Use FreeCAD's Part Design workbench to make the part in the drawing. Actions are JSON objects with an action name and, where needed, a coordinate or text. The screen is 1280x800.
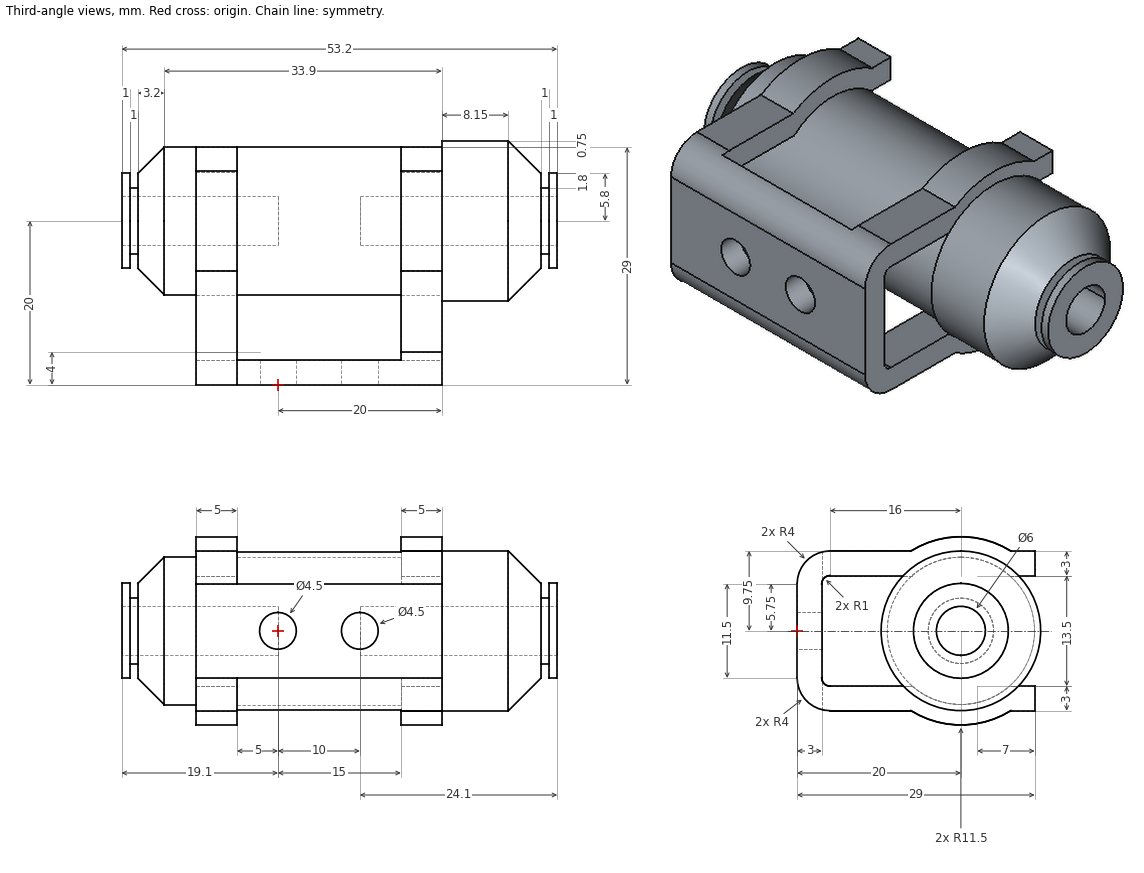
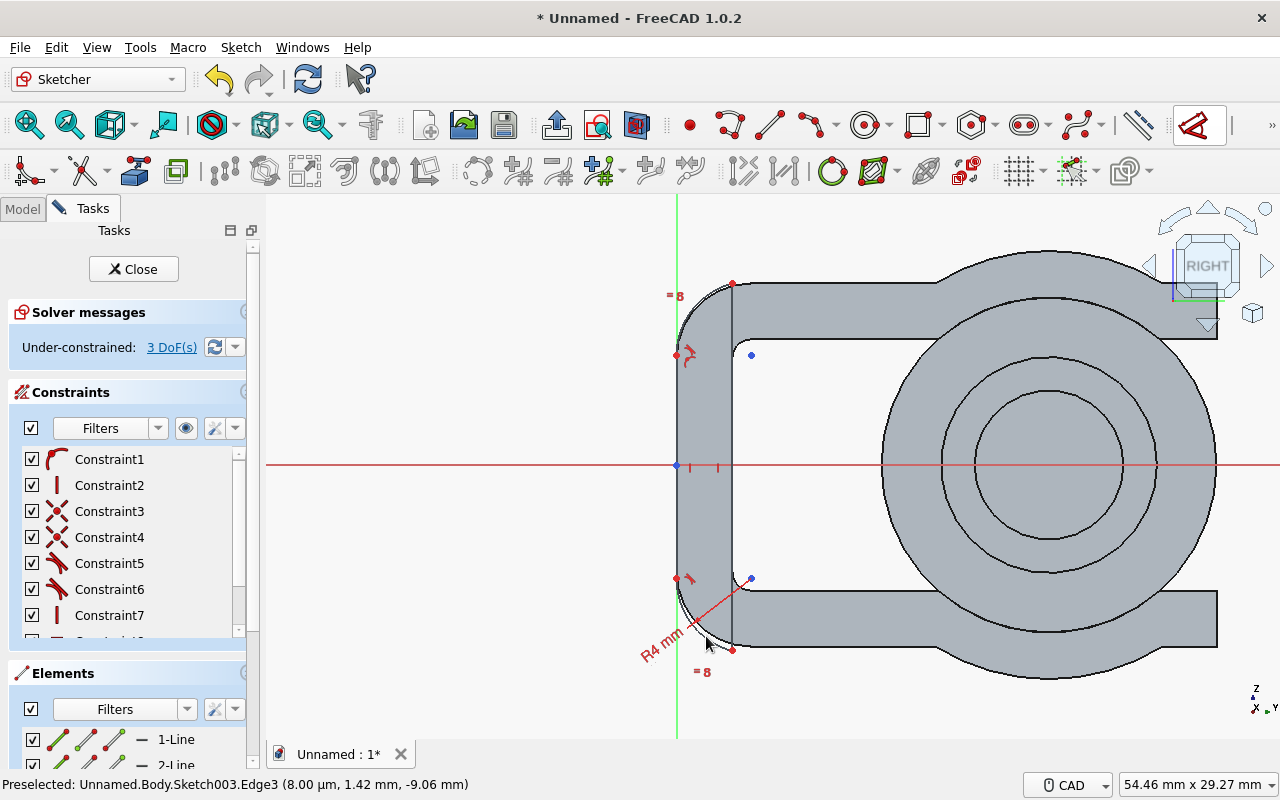
{"action": "left_click", "coordinate": [732, 651]}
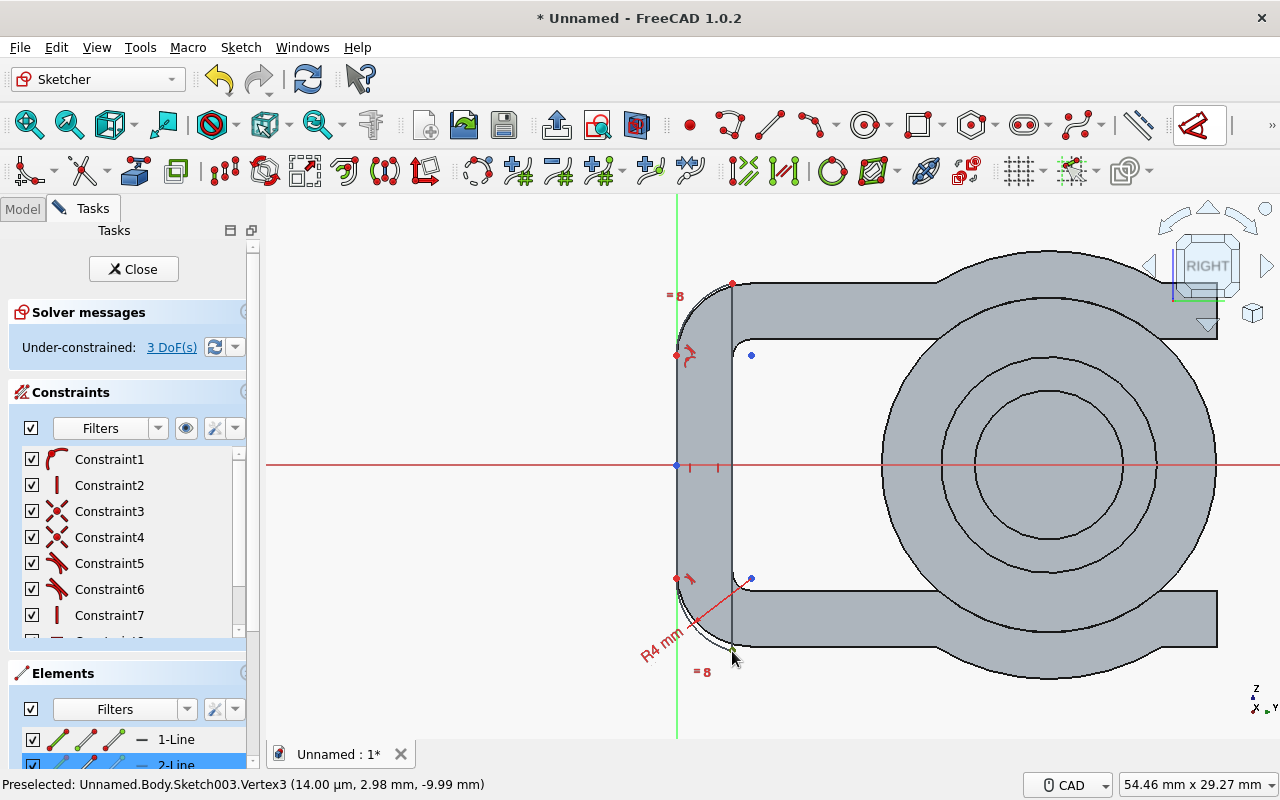
{"action": "key", "text": "l"}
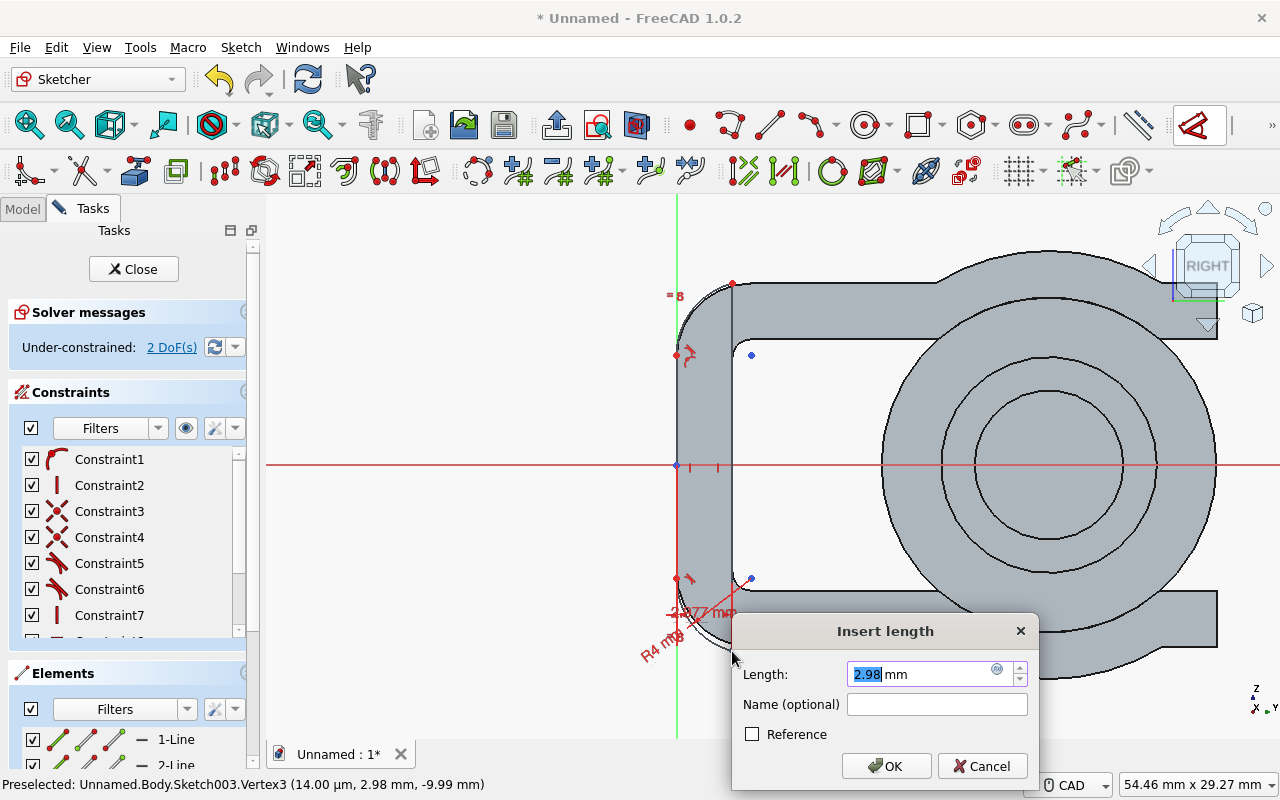
{"action": "type", "text": "3"}
{"action": "key", "text": "Return"}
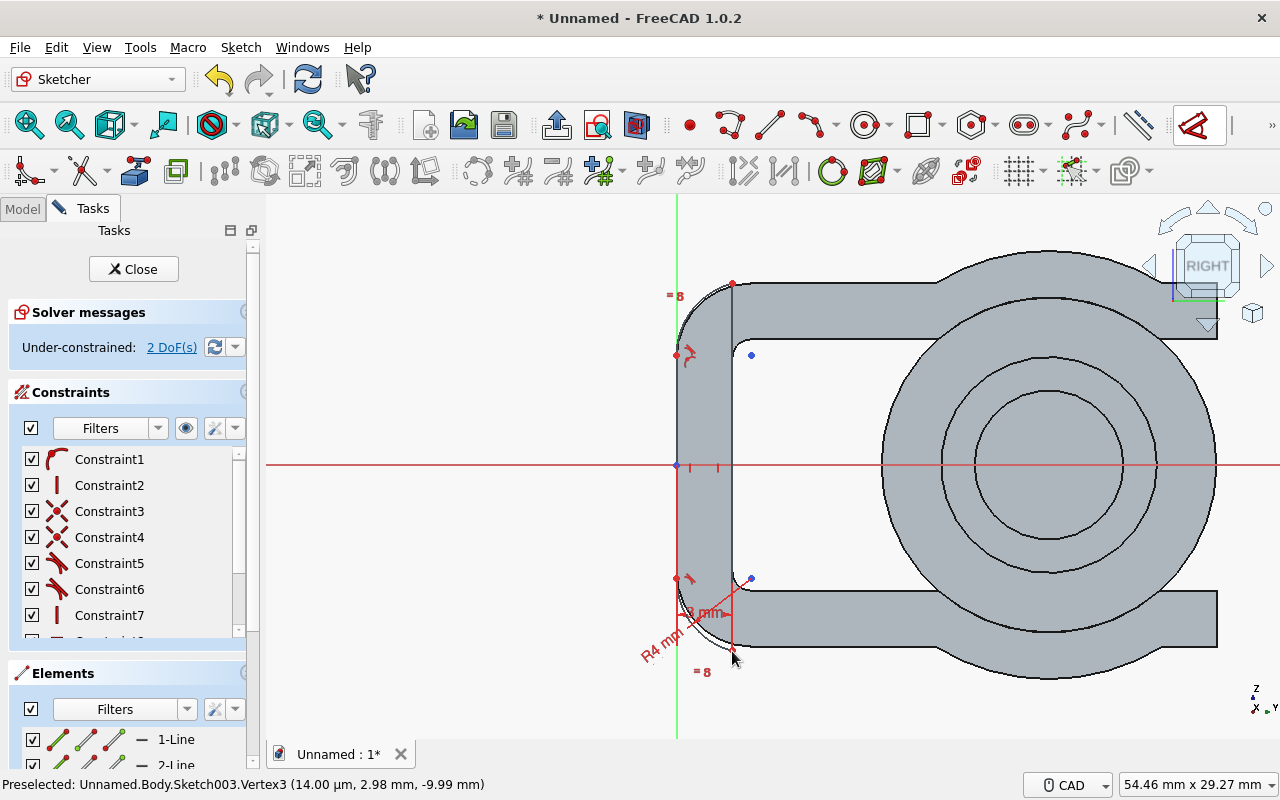
{"action": "left_click", "coordinate": [677, 423]}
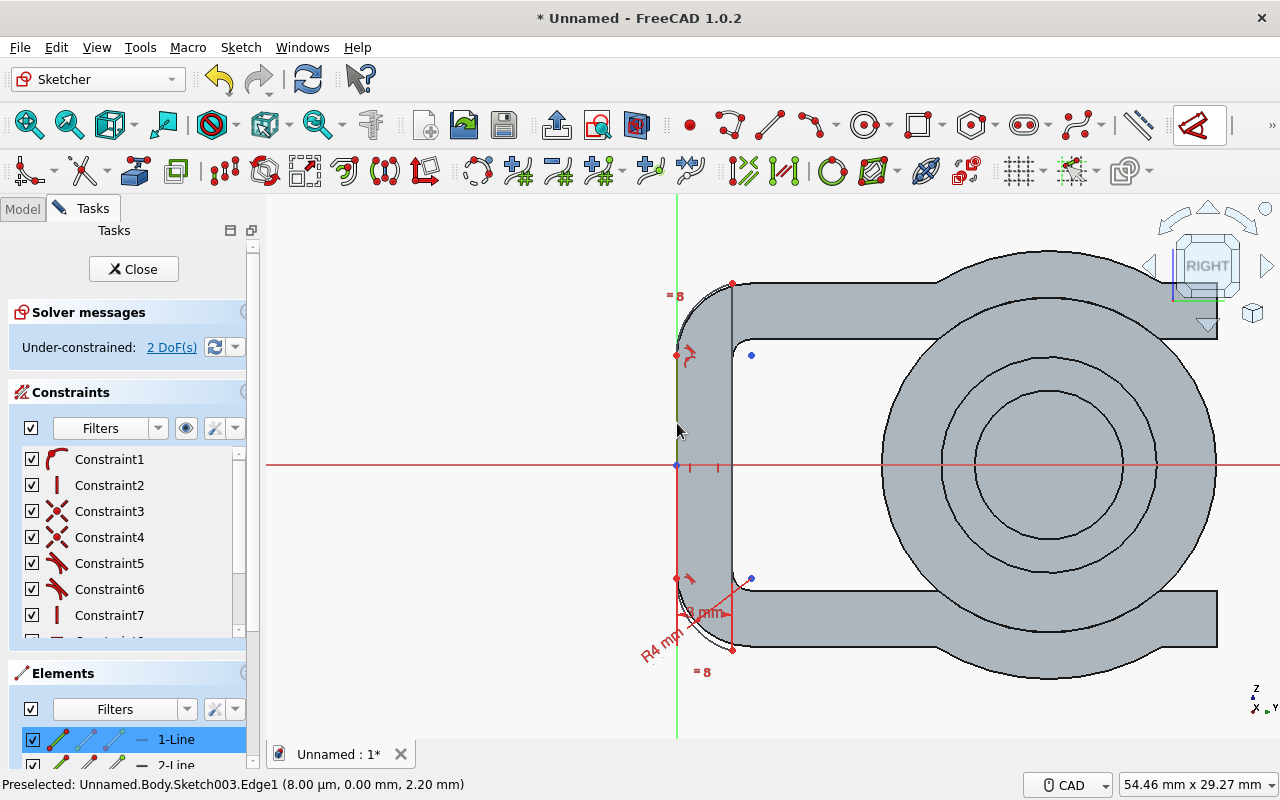
{"action": "key", "text": "i"}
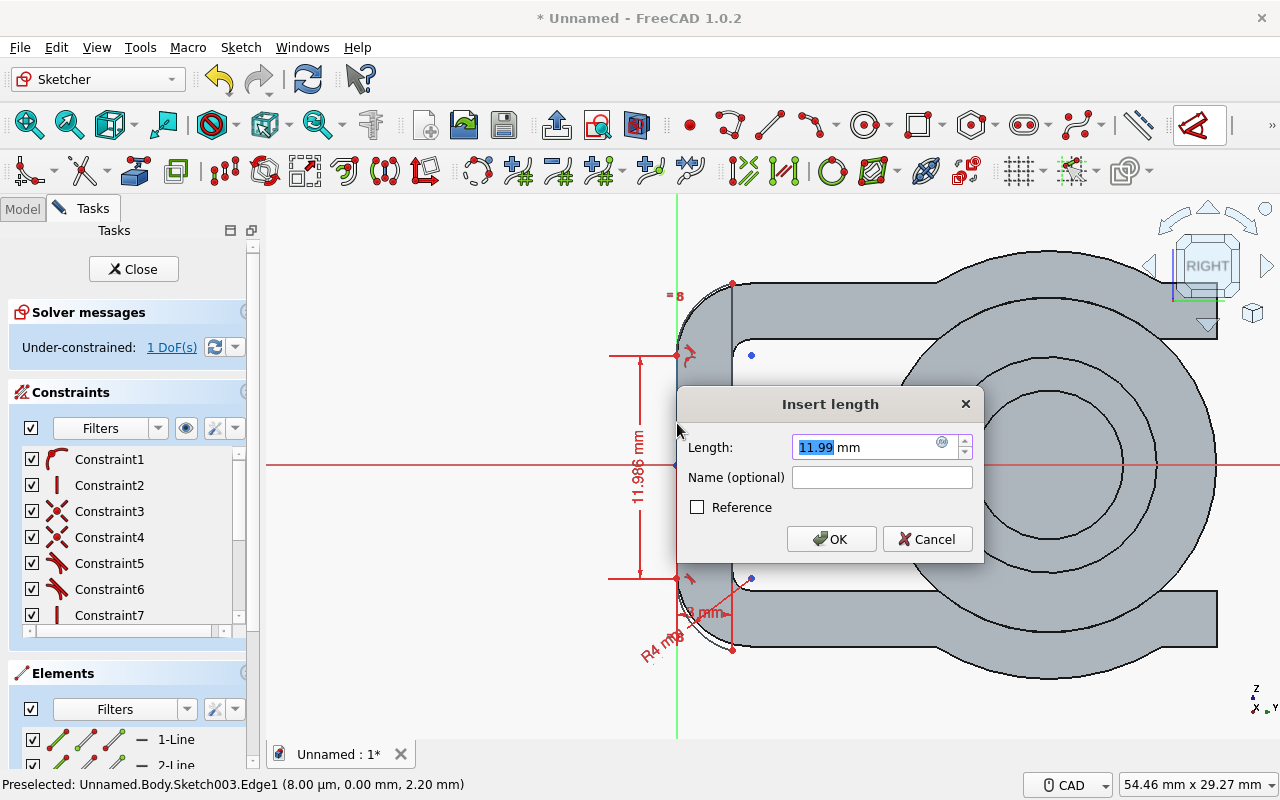
{"action": "type", "text": "11.5"}
{"action": "key", "text": "Return"}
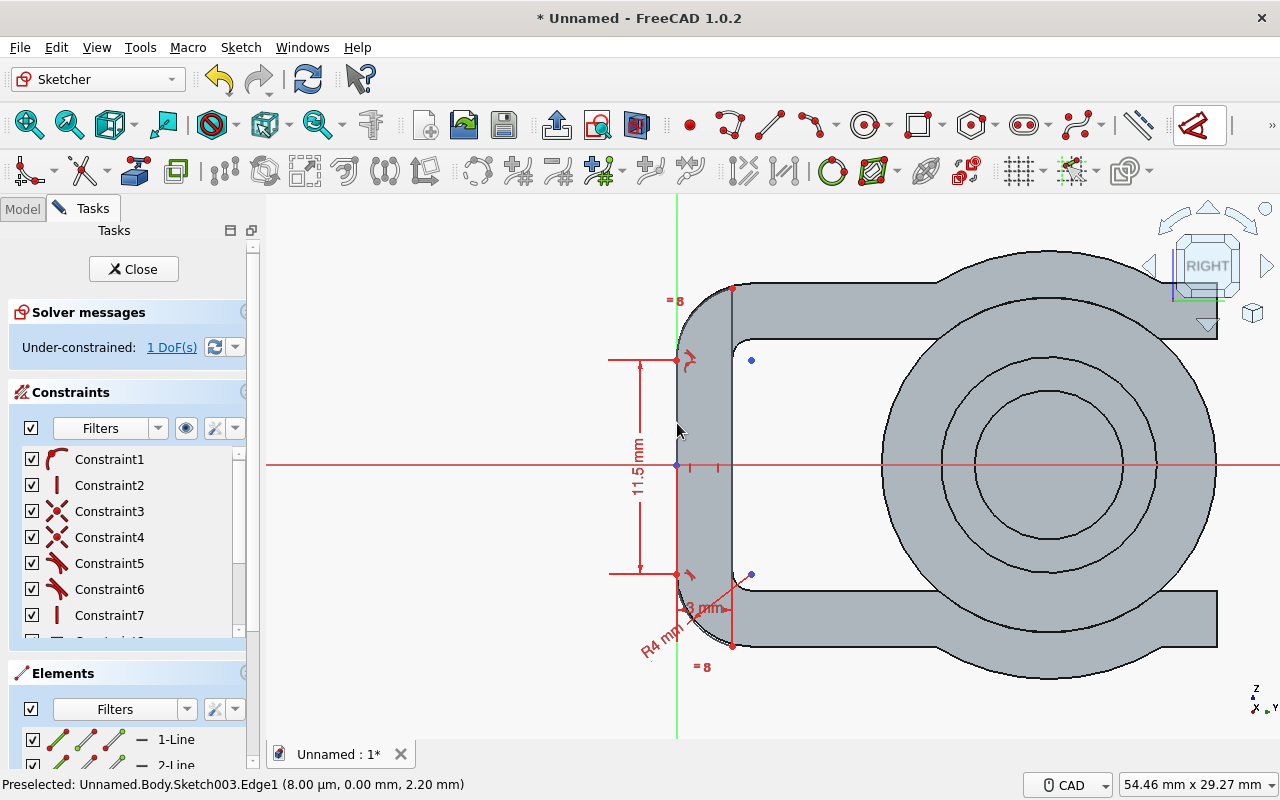
{"action": "left_click", "coordinate": [677, 360]}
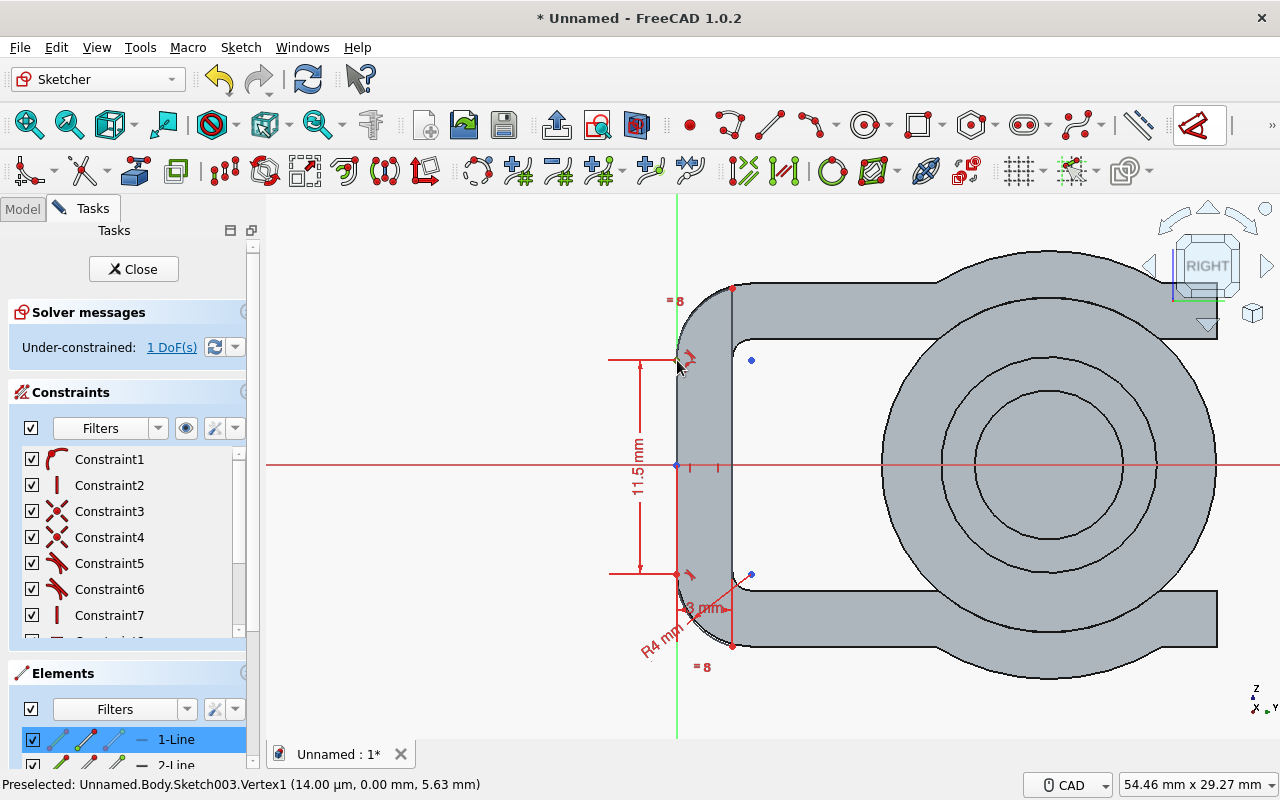
{"action": "left_click", "coordinate": [1220, 126]}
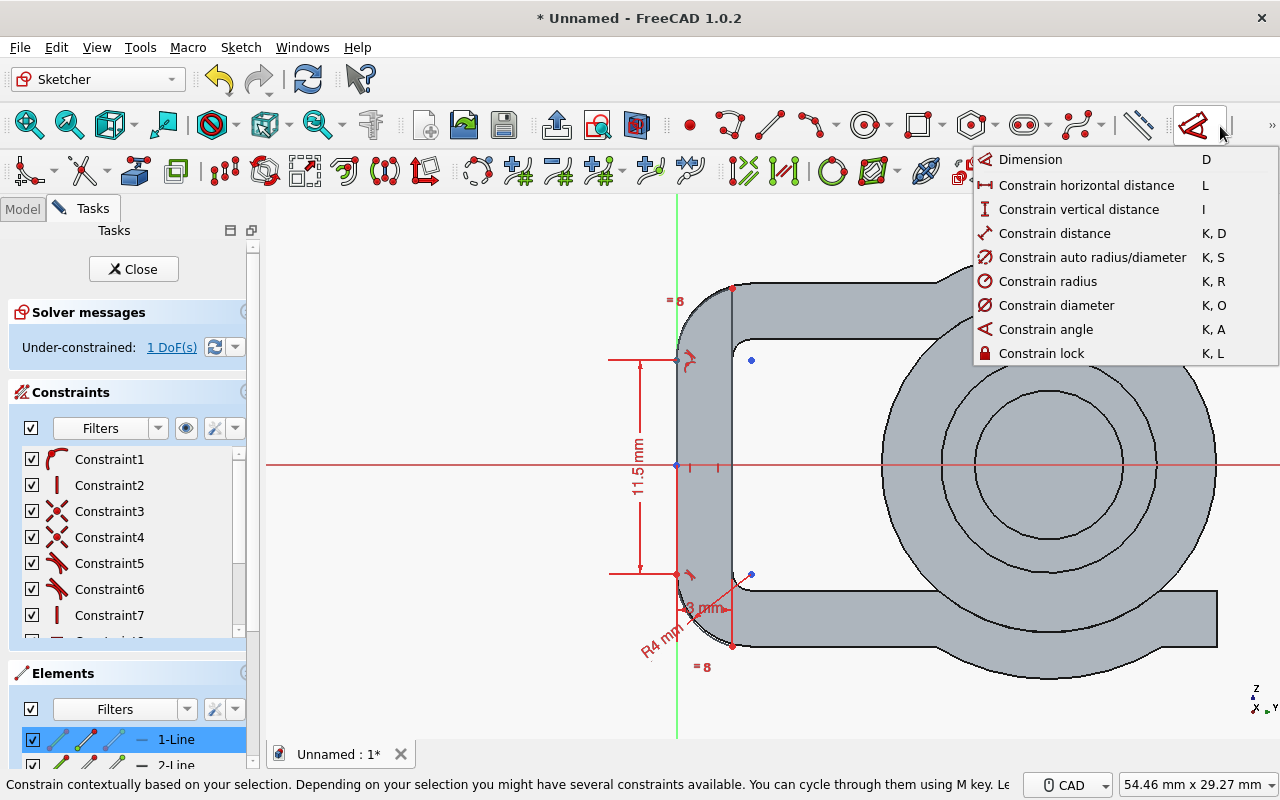
{"action": "left_click", "coordinate": [1126, 209]}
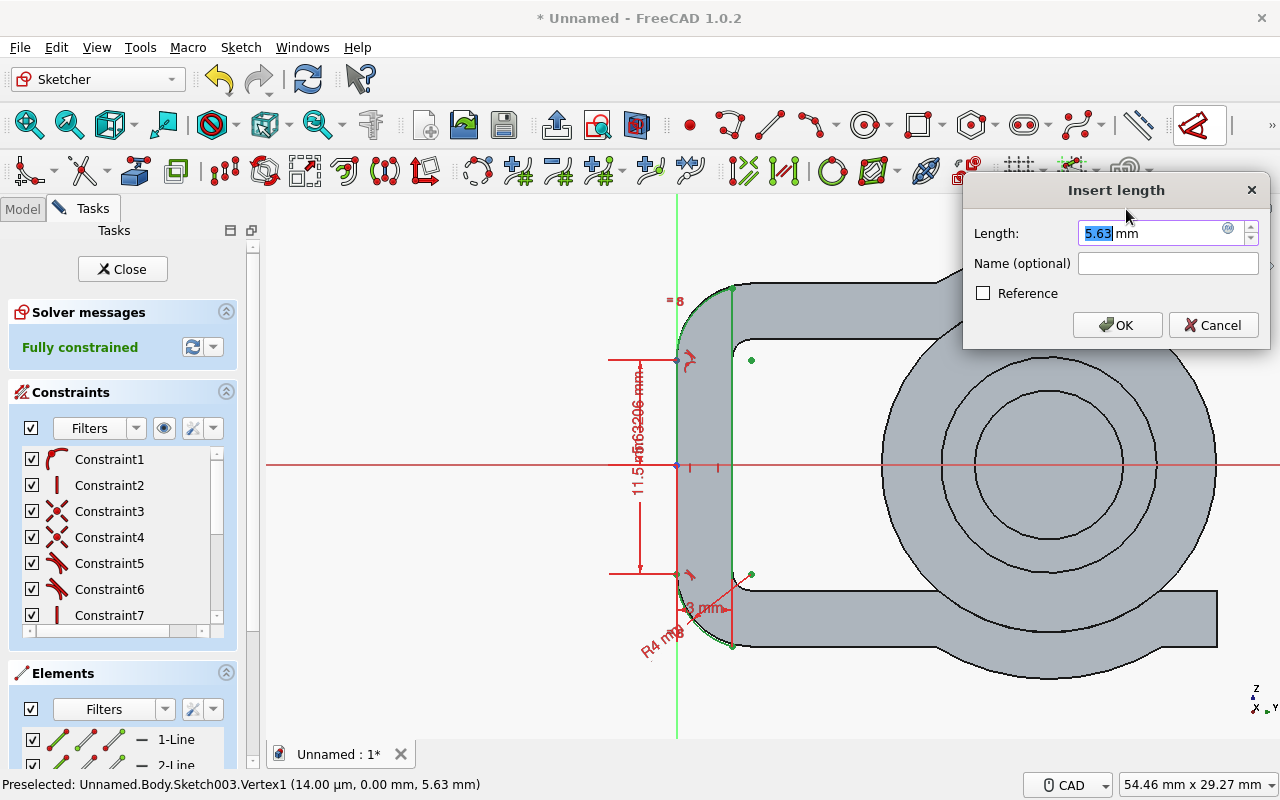
{"action": "type", "text": "5.75"}
{"action": "key", "text": "Return"}